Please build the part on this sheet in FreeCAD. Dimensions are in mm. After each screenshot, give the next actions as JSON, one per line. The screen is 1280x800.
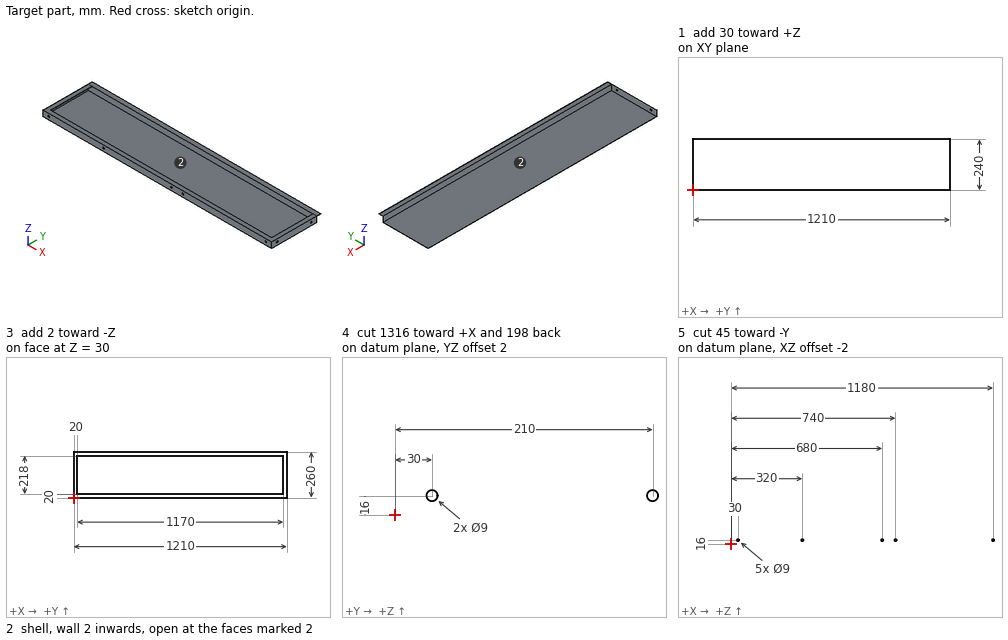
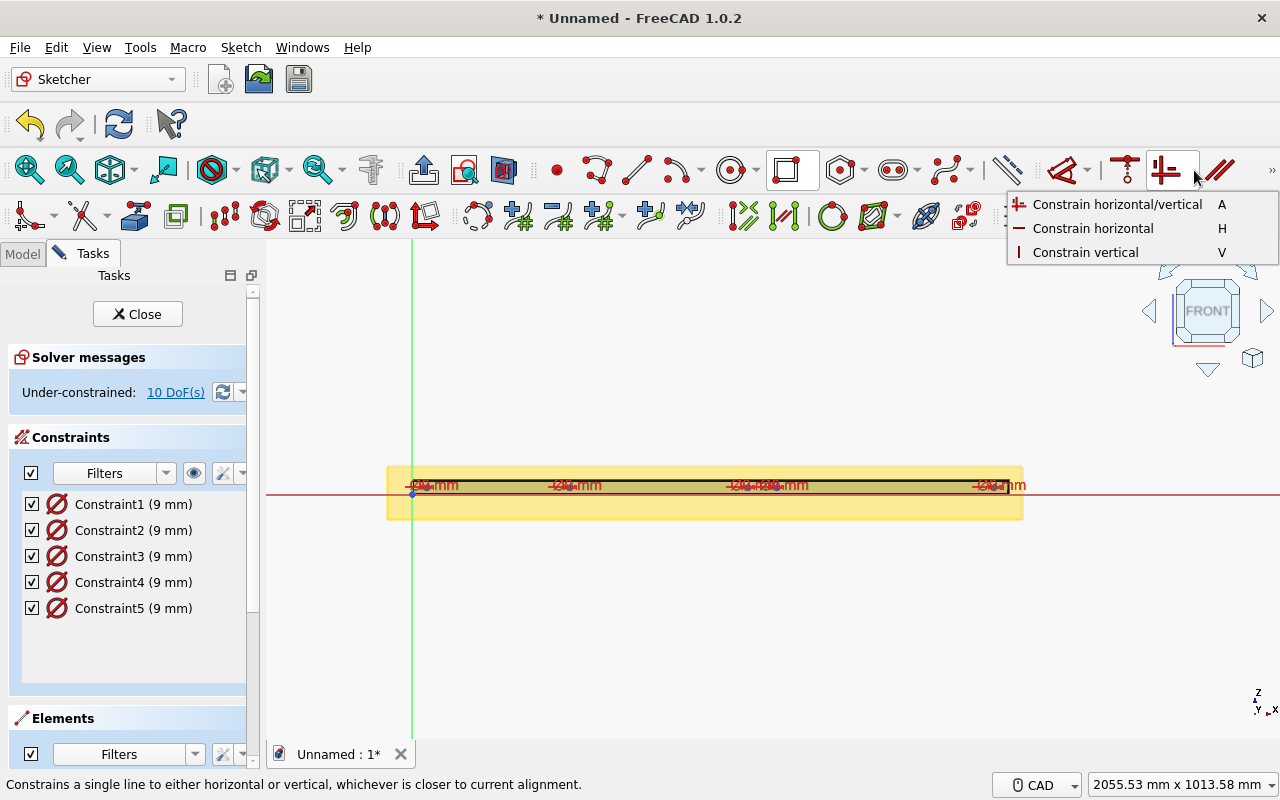
{"action": "left_click", "coordinate": [1143, 228]}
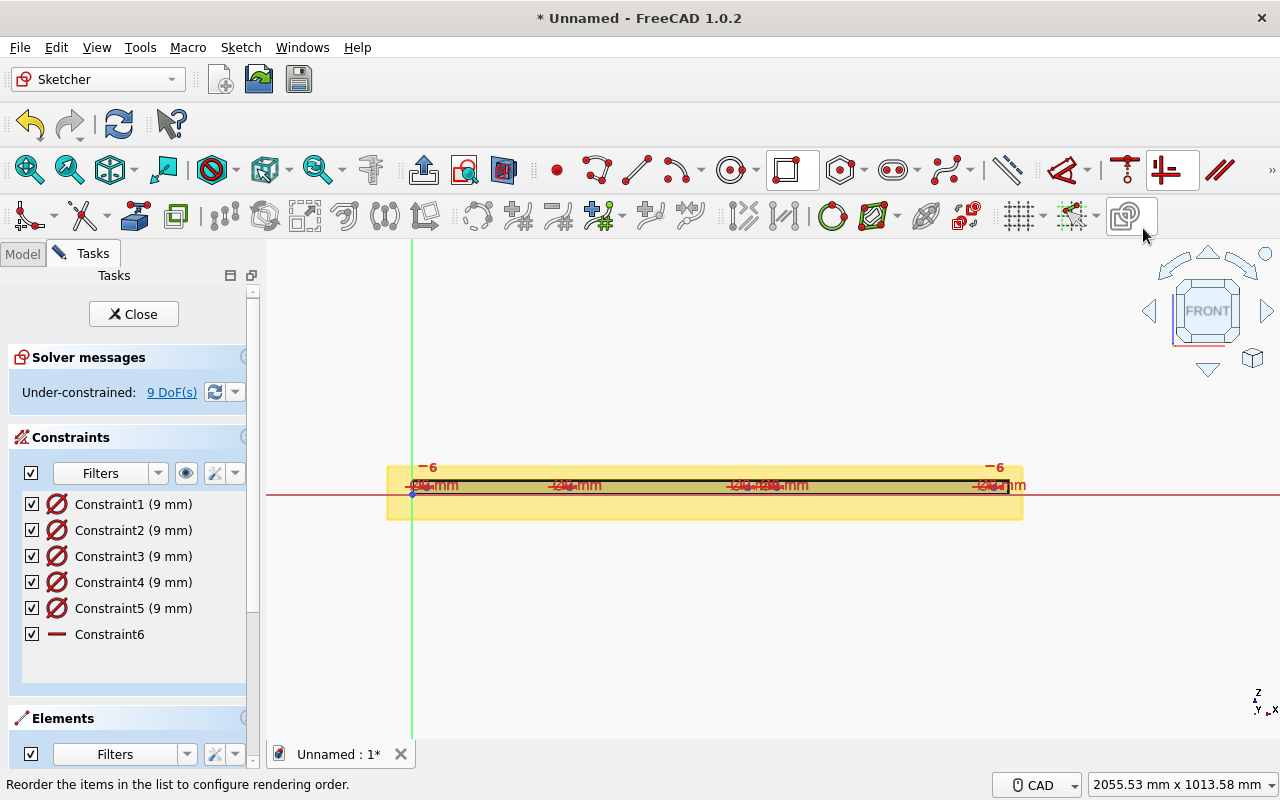
{"action": "left_click", "coordinate": [995, 487]}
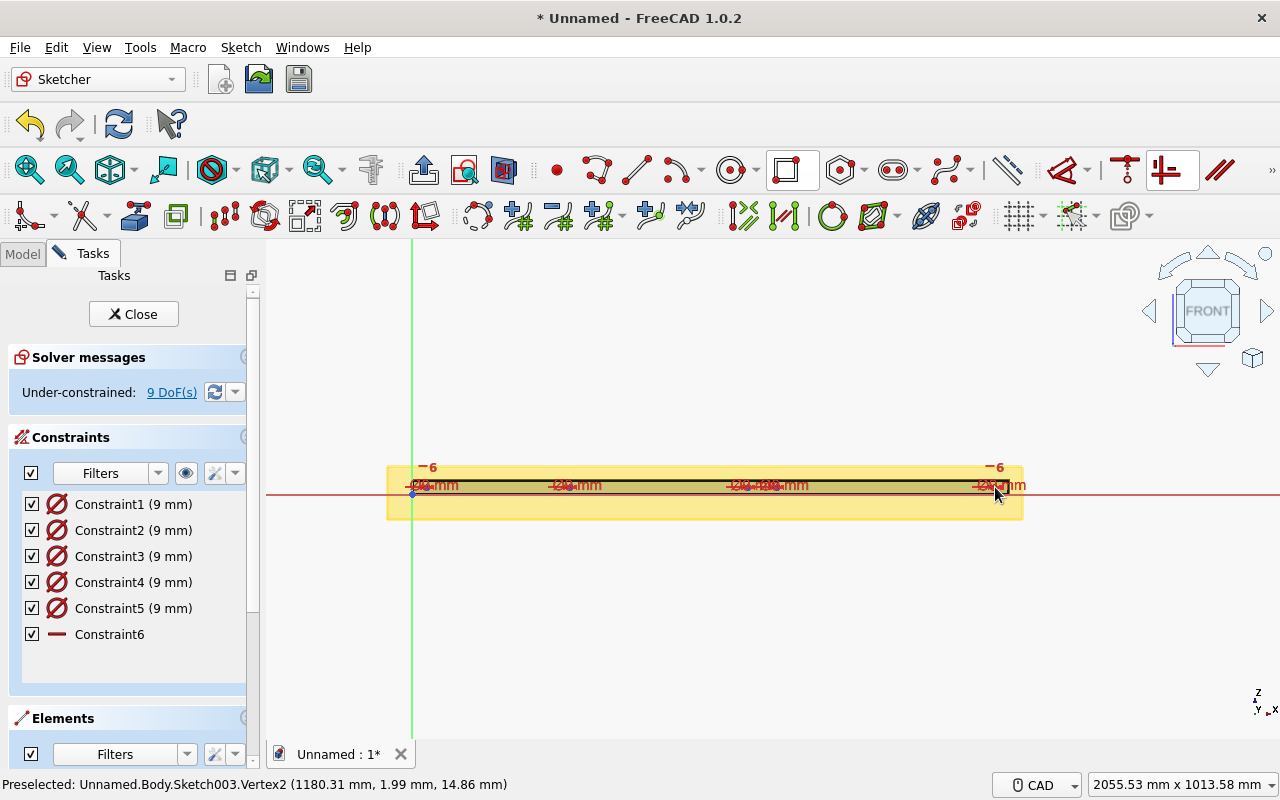
{"action": "left_click", "coordinate": [748, 487]}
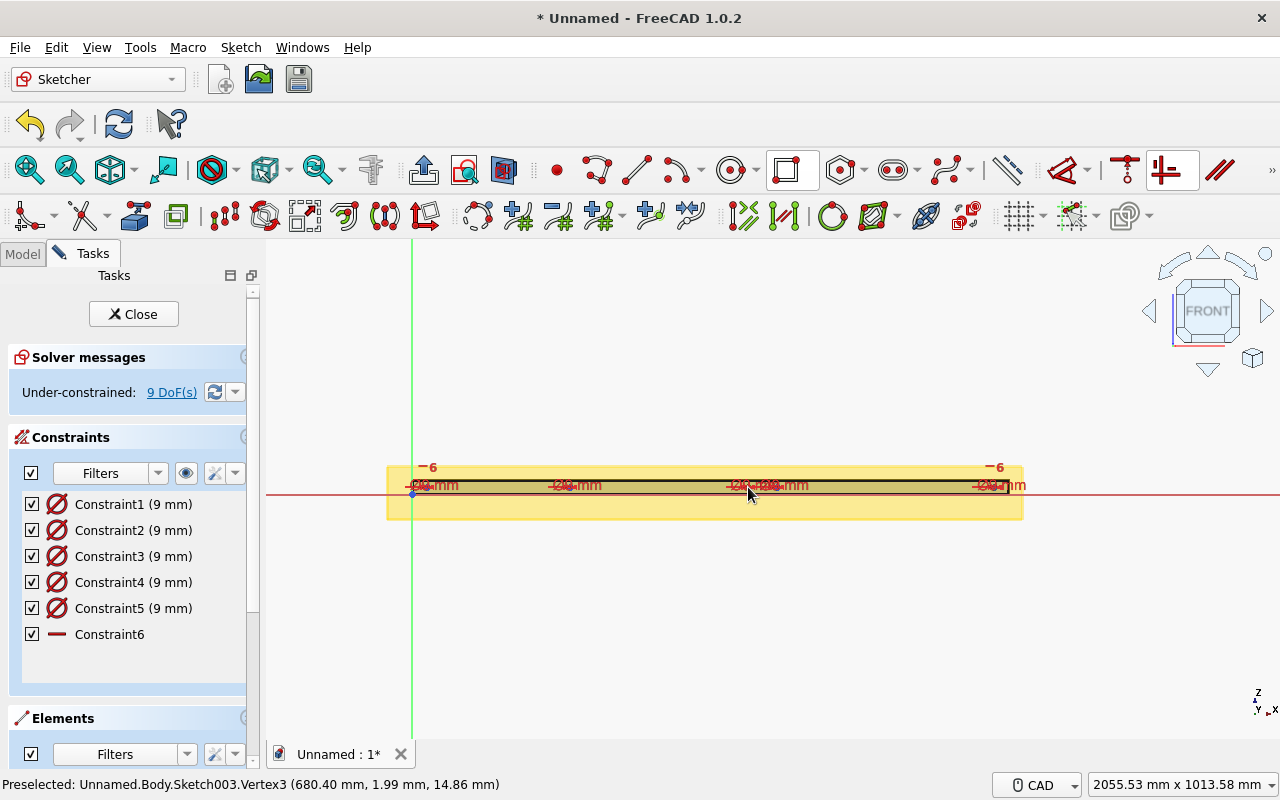
{"action": "left_click", "coordinate": [1194, 170]}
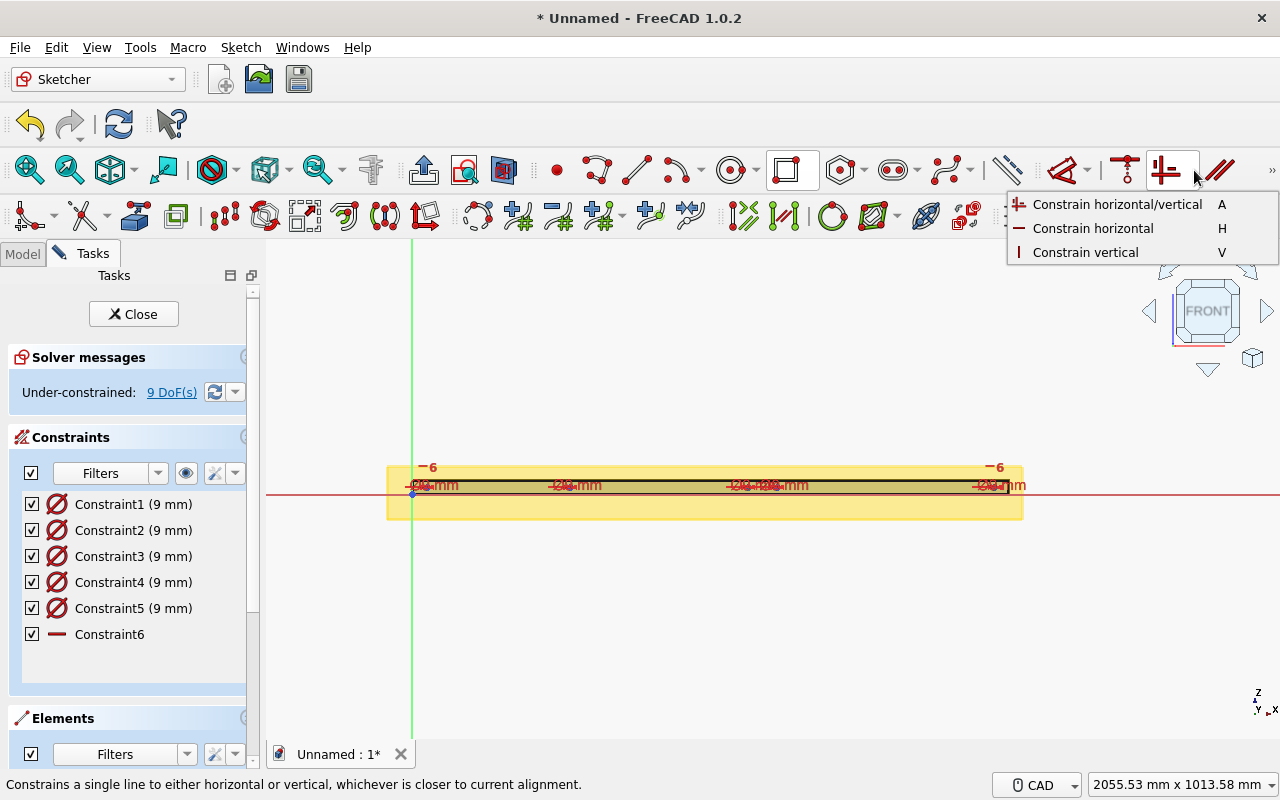
{"action": "left_click", "coordinate": [1143, 228]}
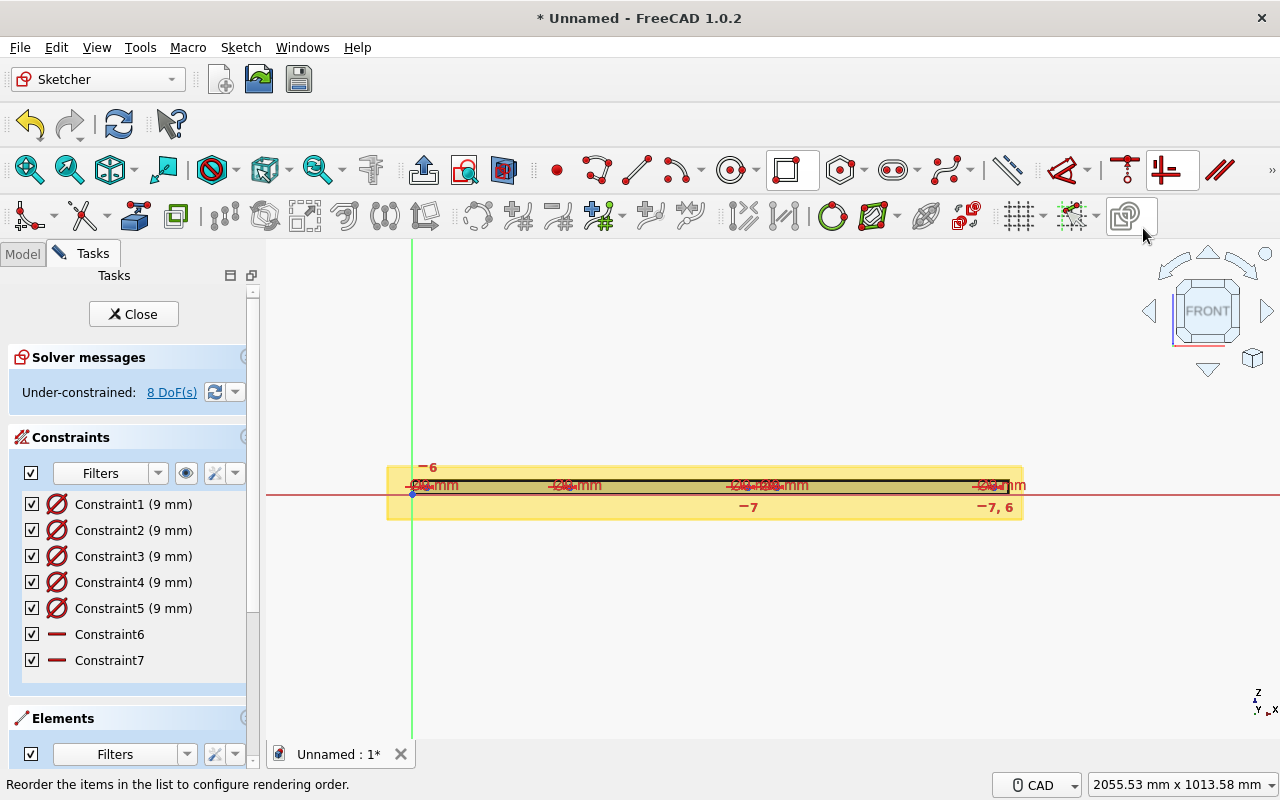
{"action": "left_click", "coordinate": [427, 487]}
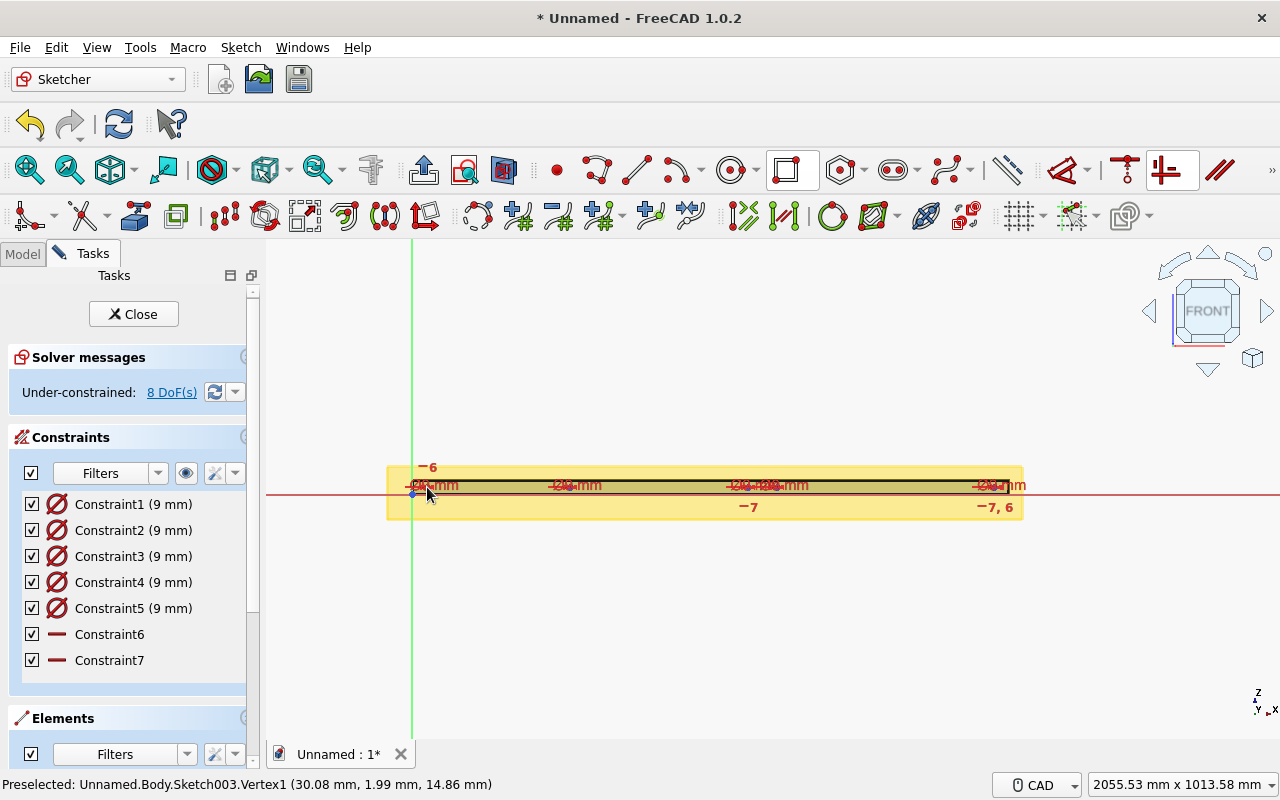
{"action": "left_click", "coordinate": [570, 487]}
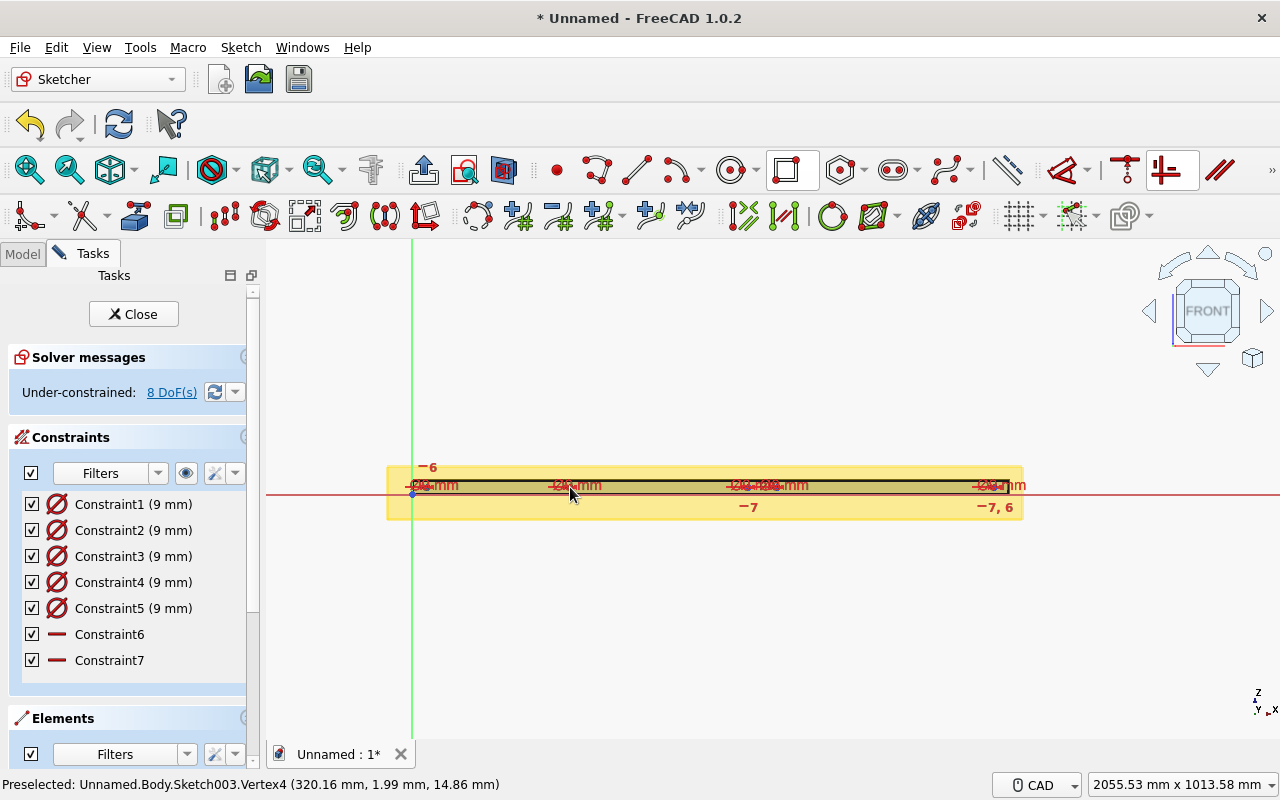
{"action": "key", "text": "h"}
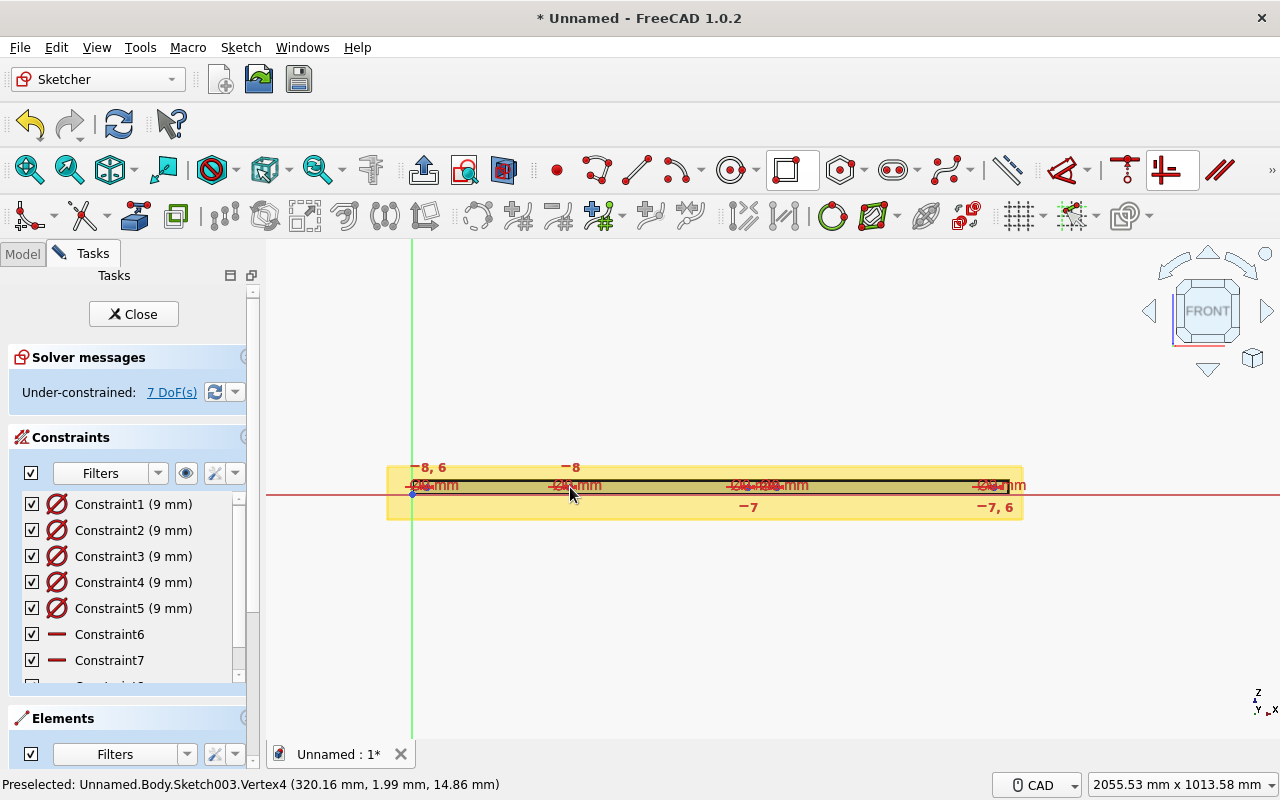
{"action": "left_click", "coordinate": [748, 487]}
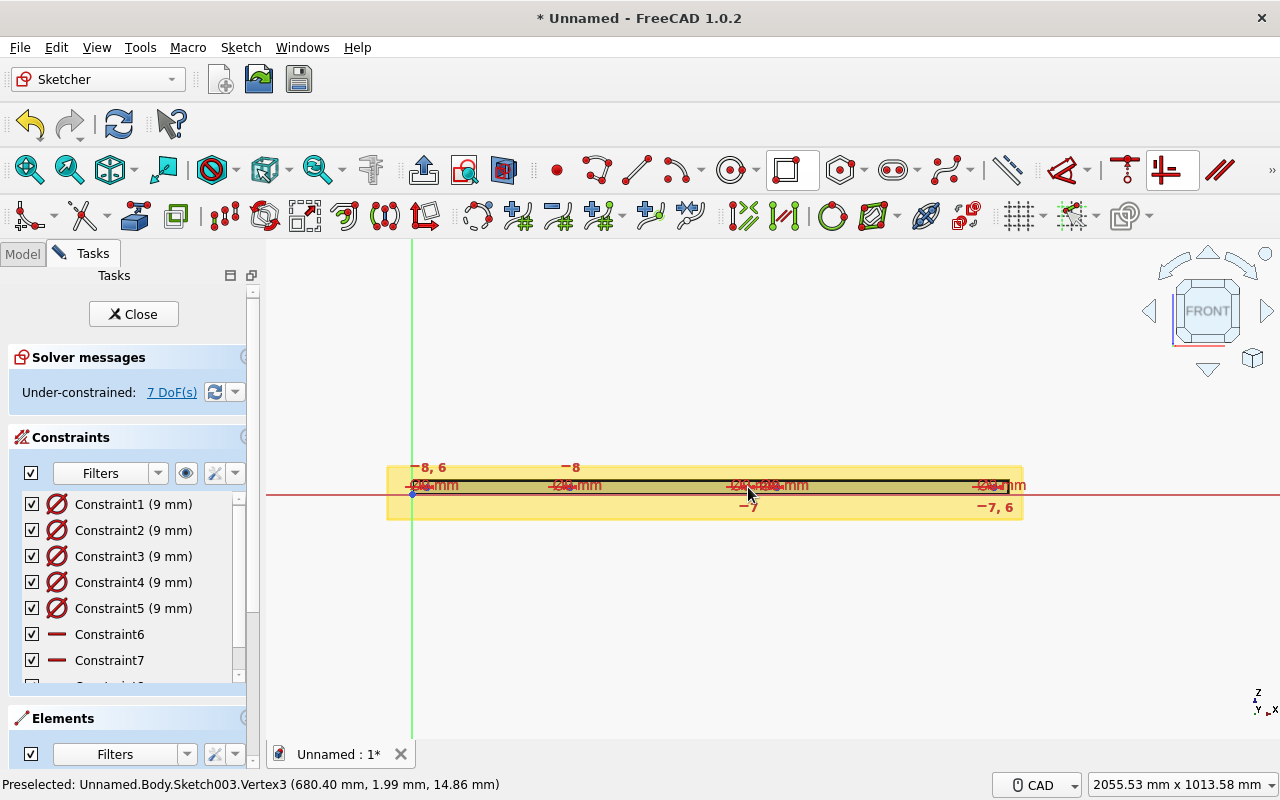
{"action": "left_click", "coordinate": [777, 487]}